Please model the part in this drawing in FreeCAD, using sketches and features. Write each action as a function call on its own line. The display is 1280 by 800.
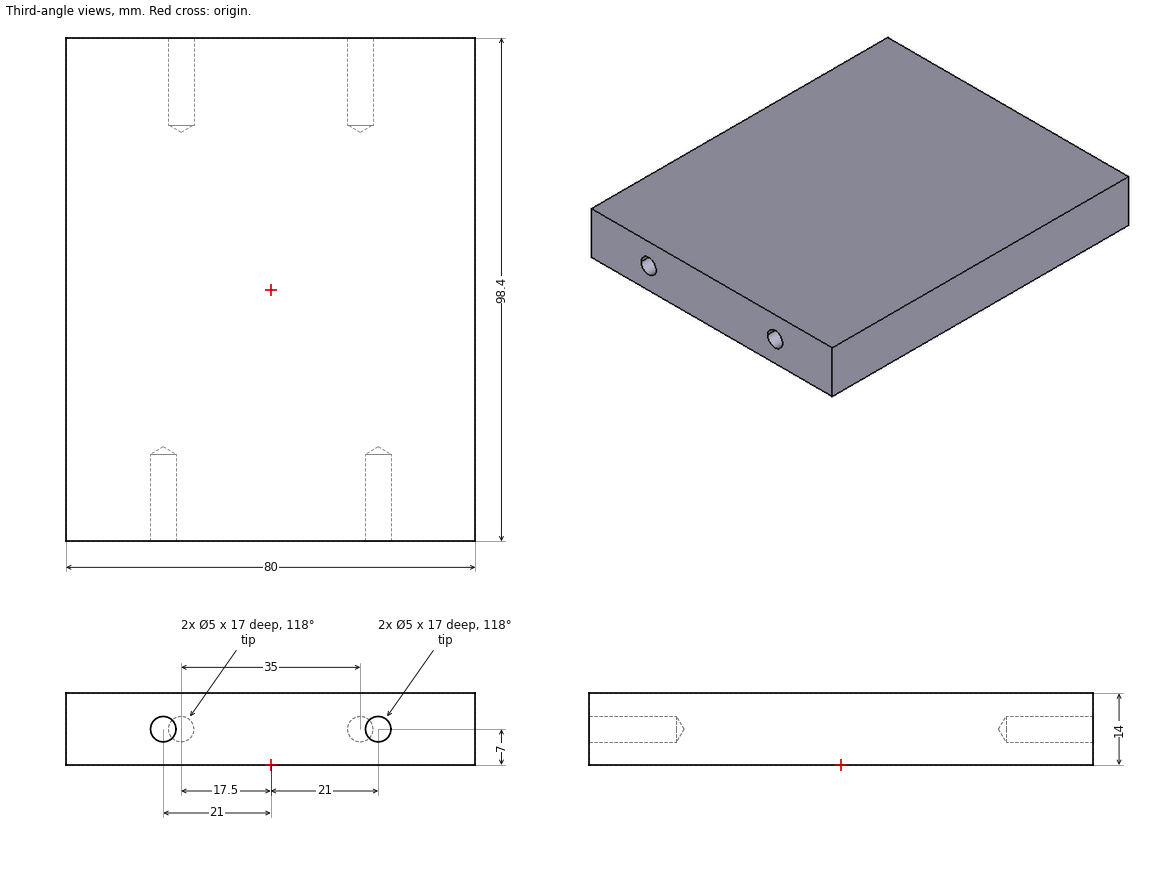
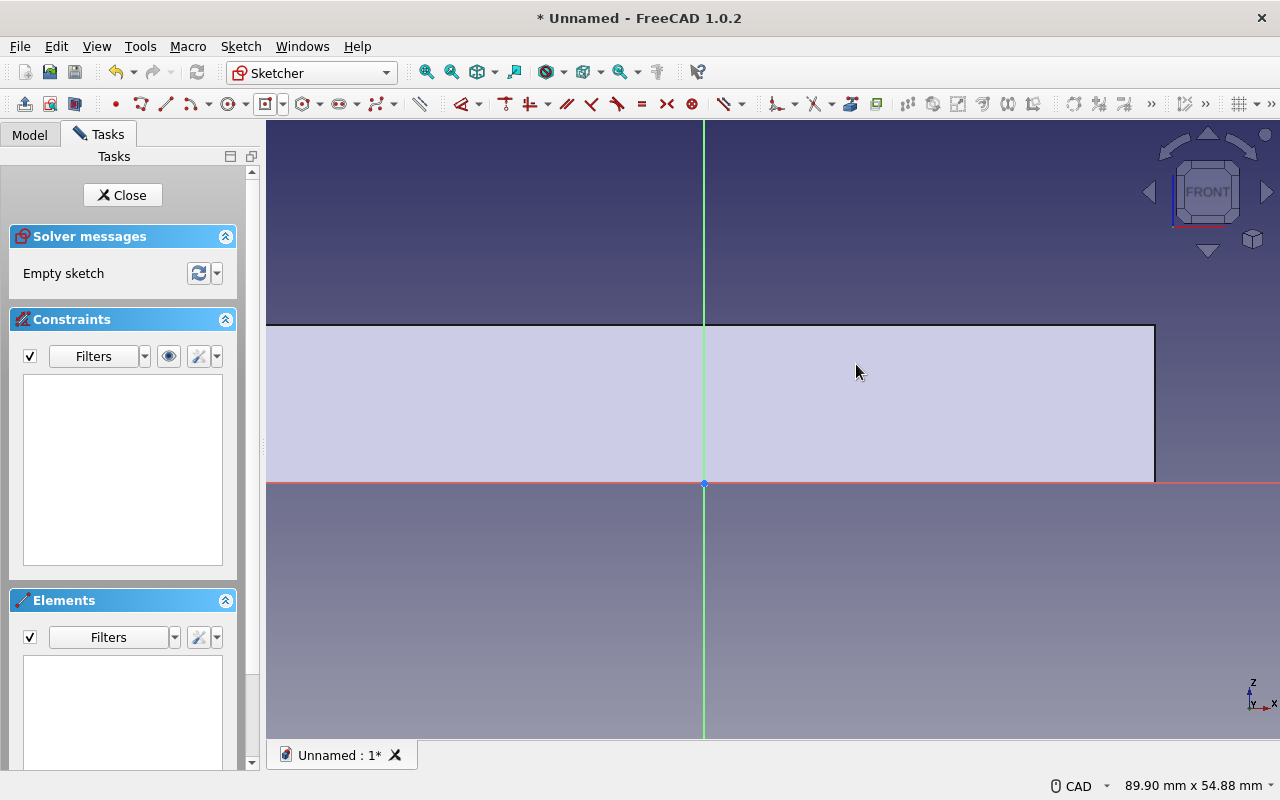
click(228, 104)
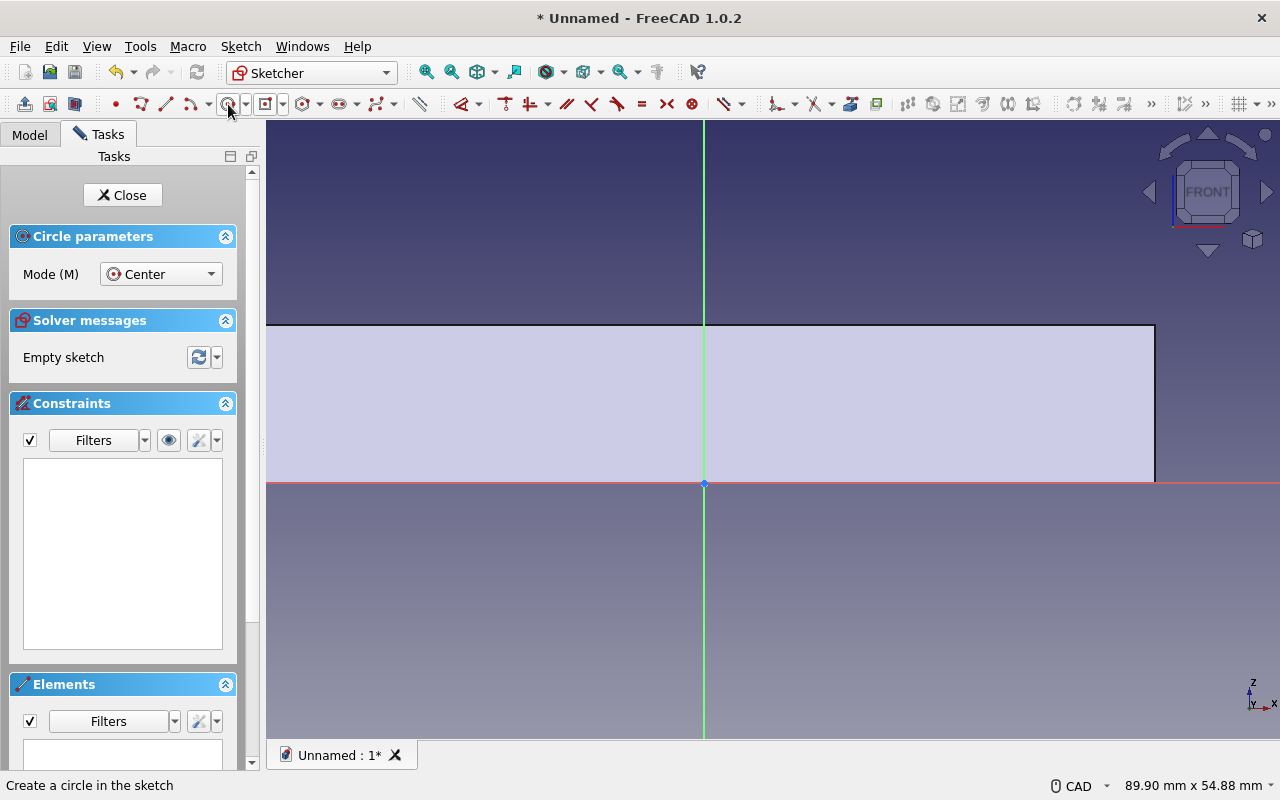
click(941, 404)
click(961, 384)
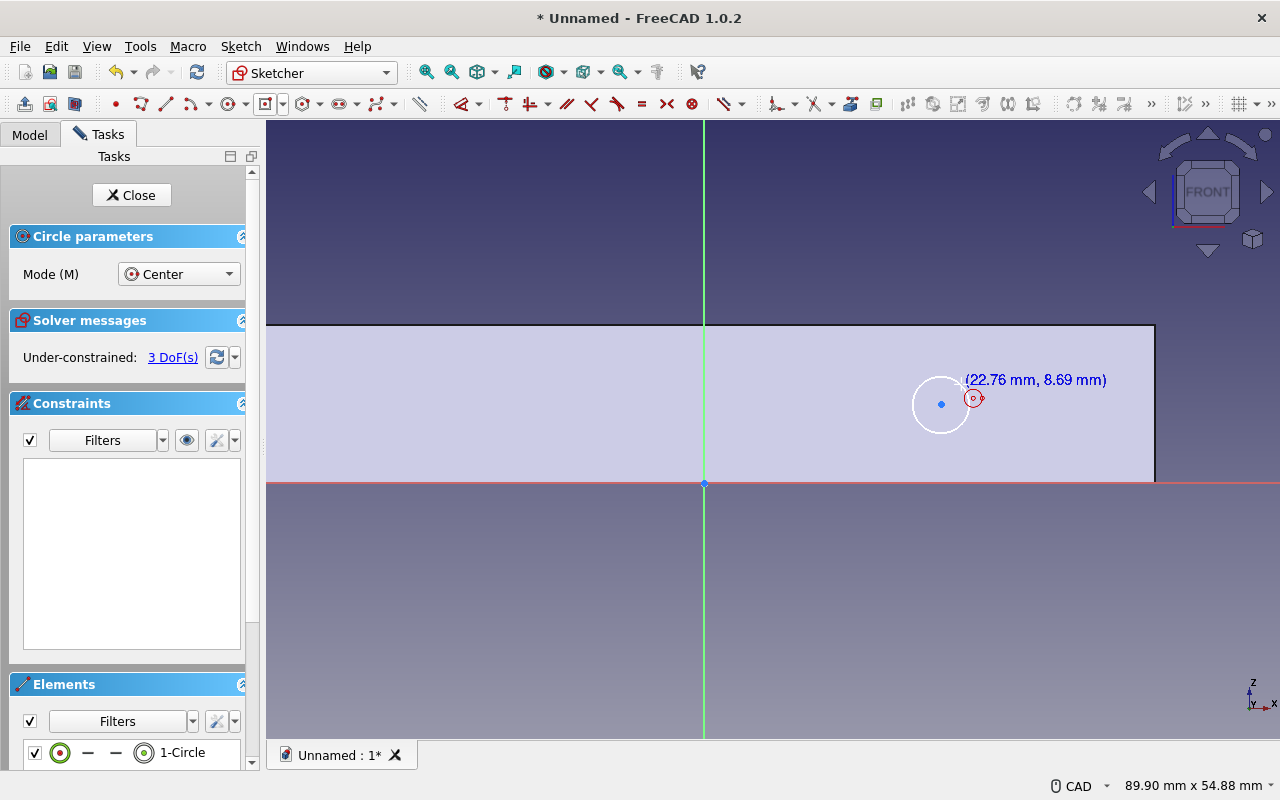
click(467, 404)
click(487, 384)
key(Escape)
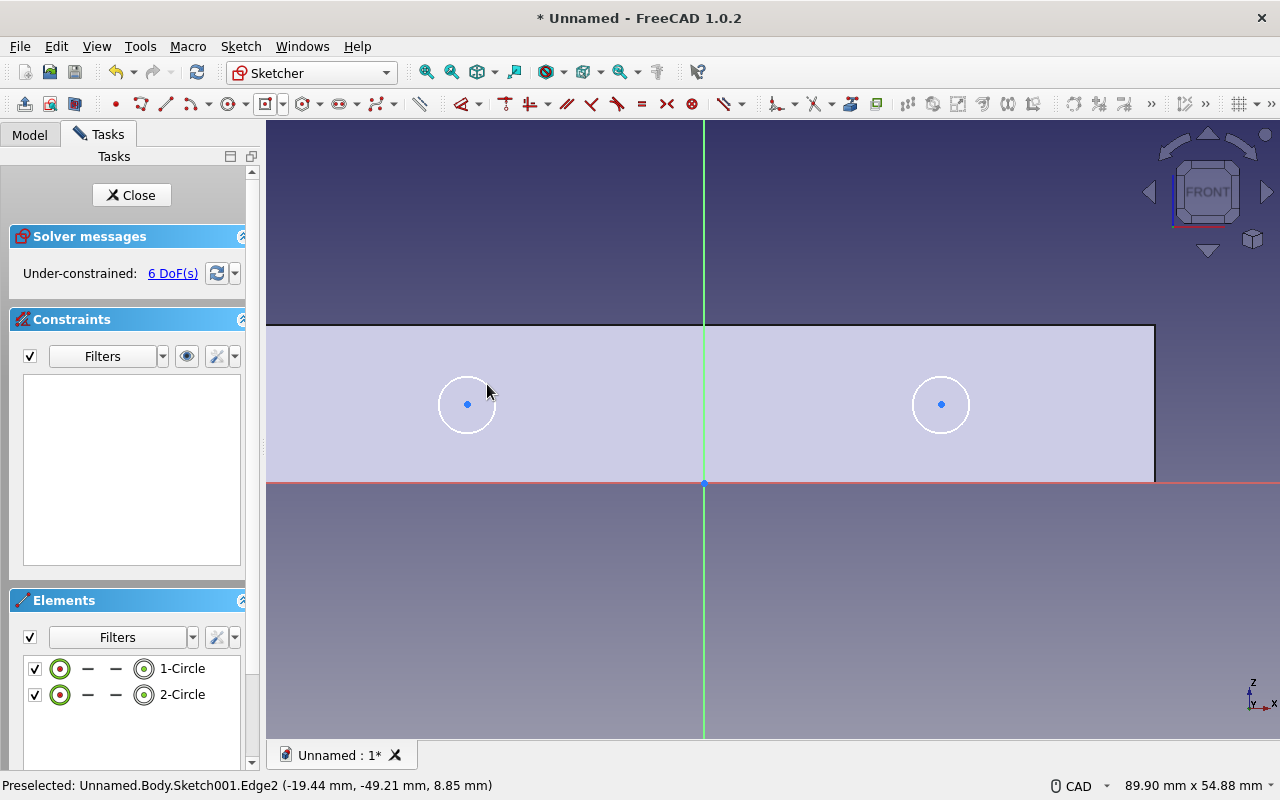
click(961, 385)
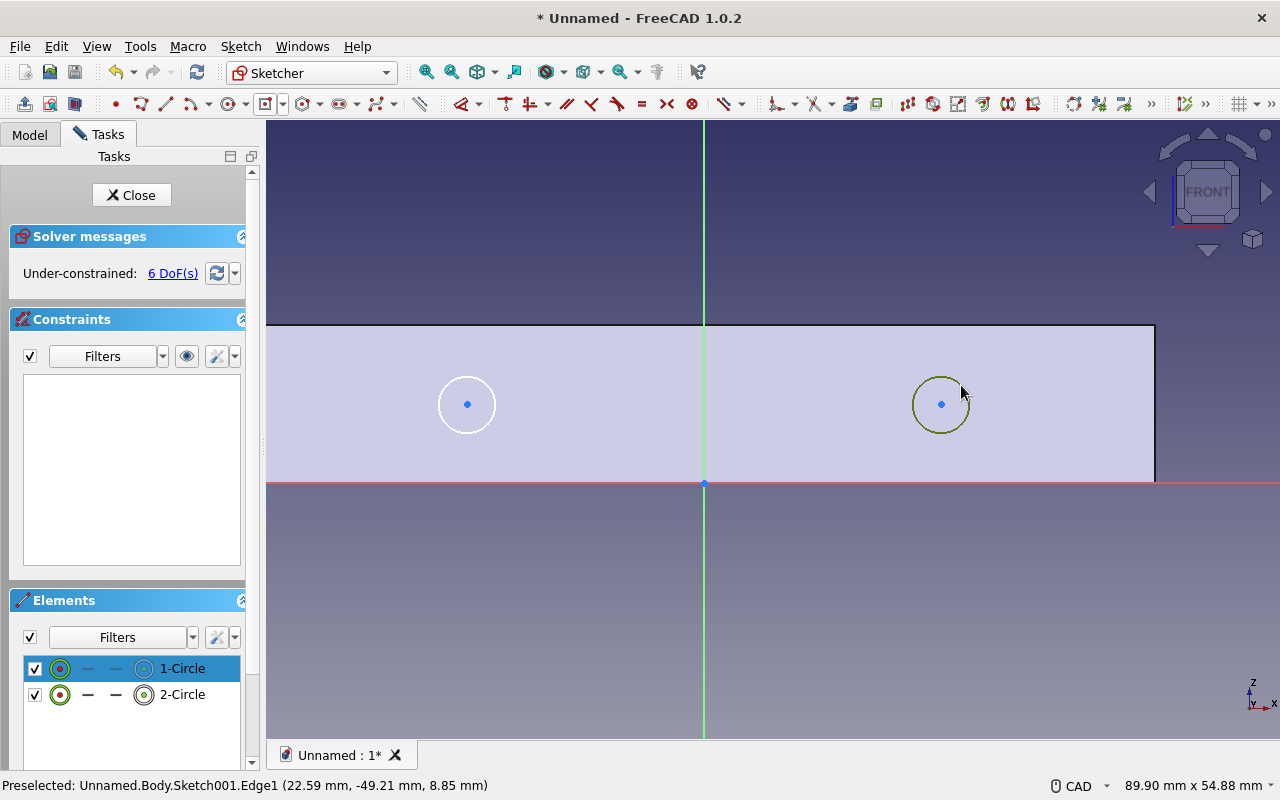
click(487, 385)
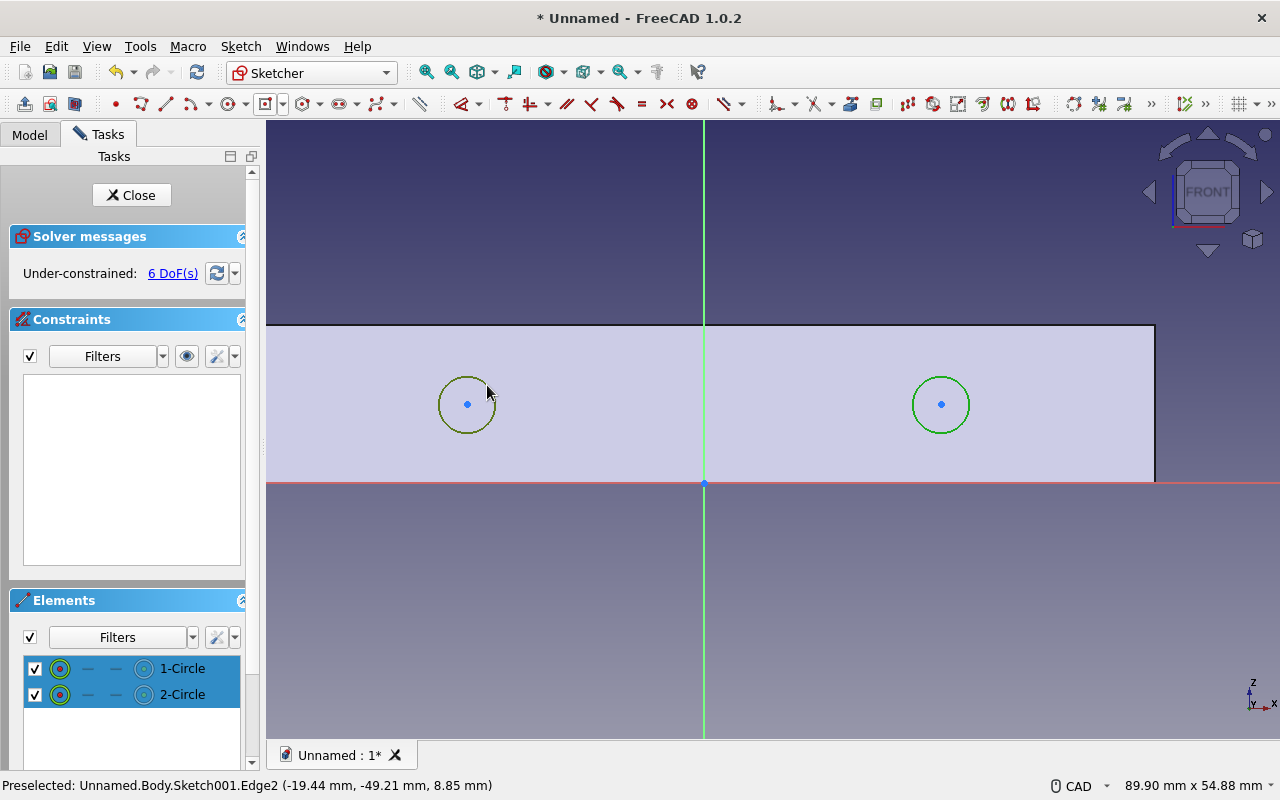
click(642, 104)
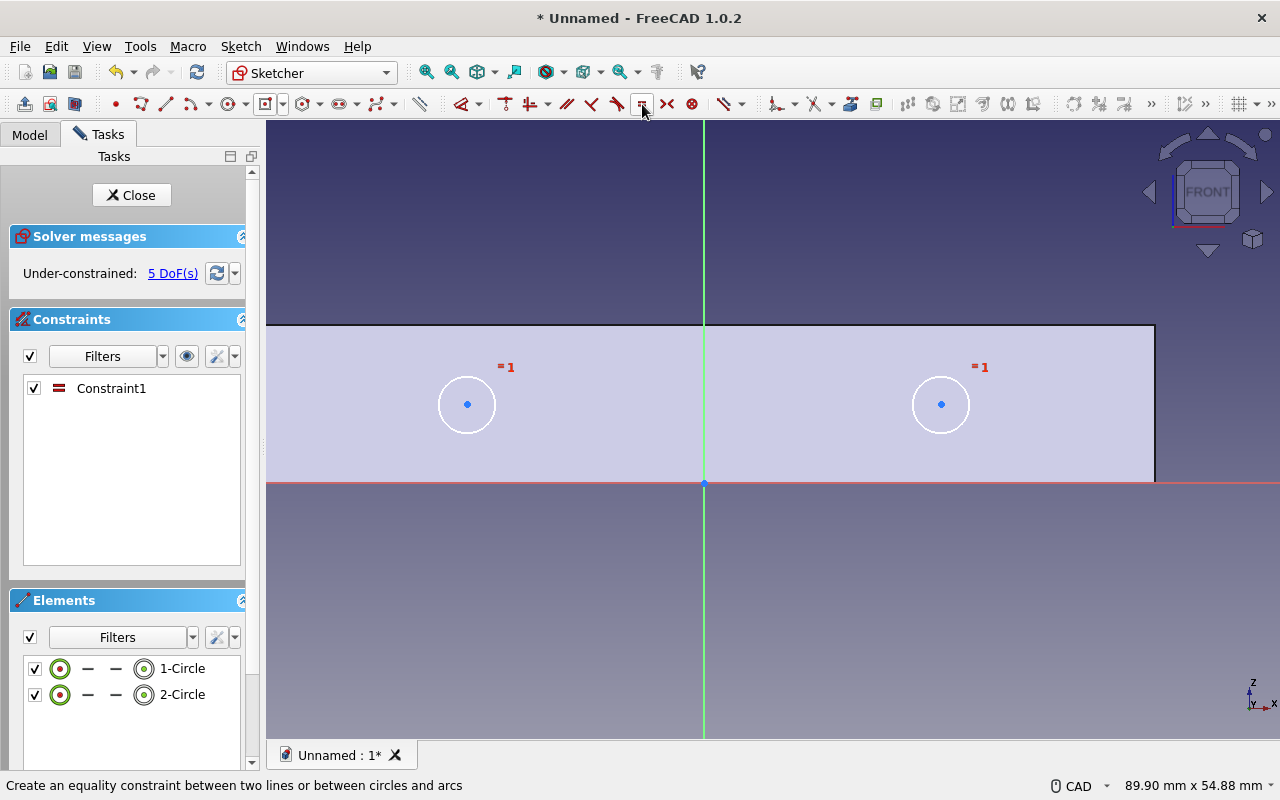
click(941, 405)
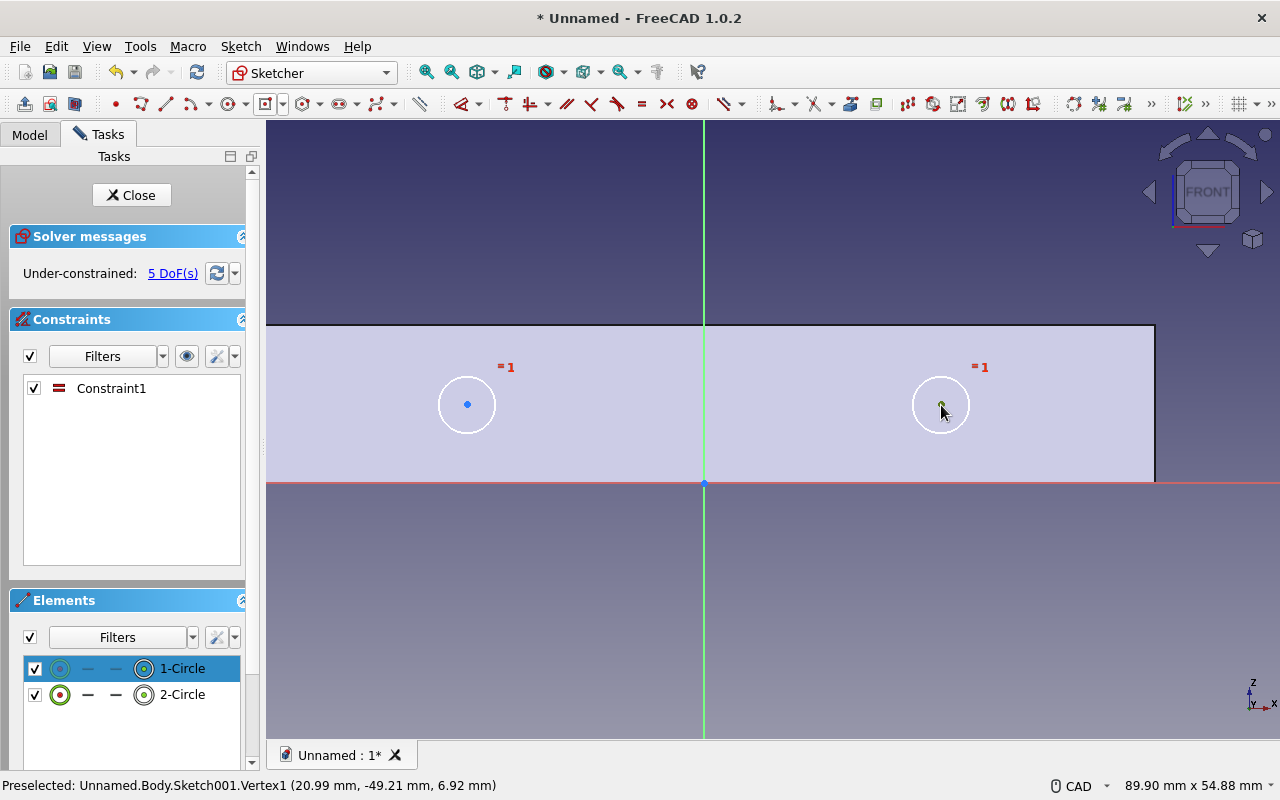
click(467, 405)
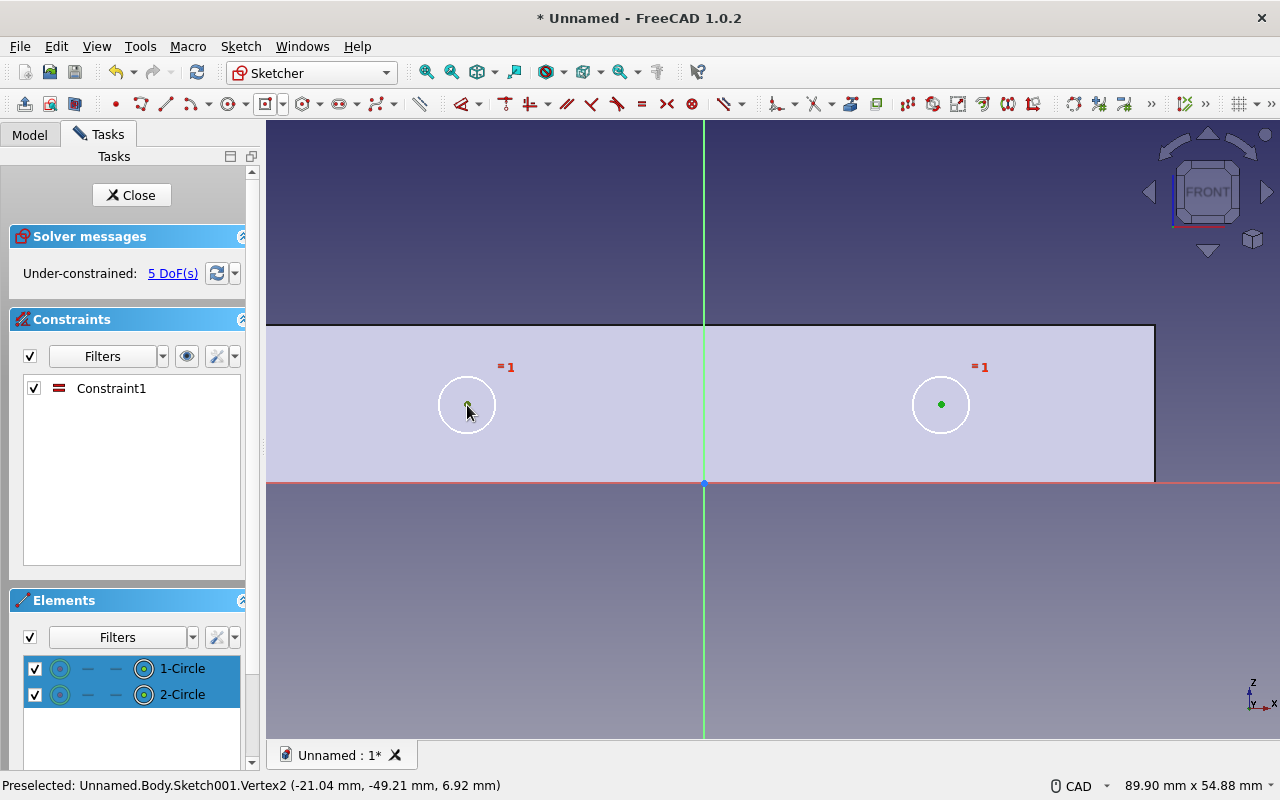
key(h)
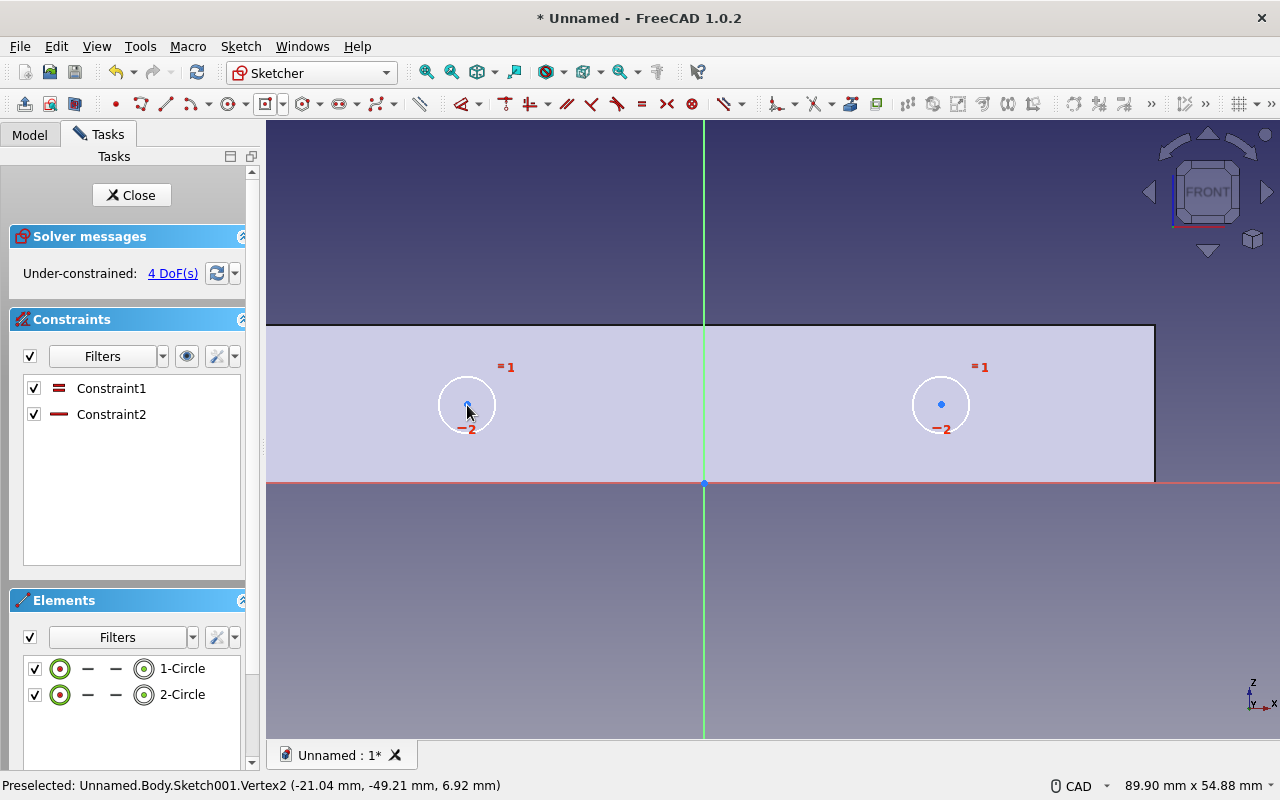
click(460, 104)